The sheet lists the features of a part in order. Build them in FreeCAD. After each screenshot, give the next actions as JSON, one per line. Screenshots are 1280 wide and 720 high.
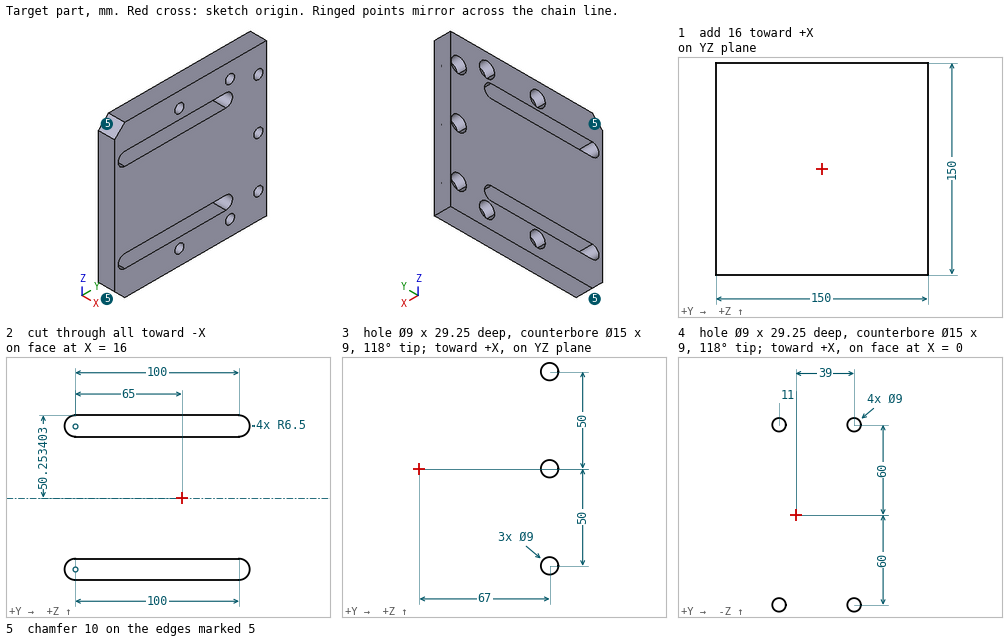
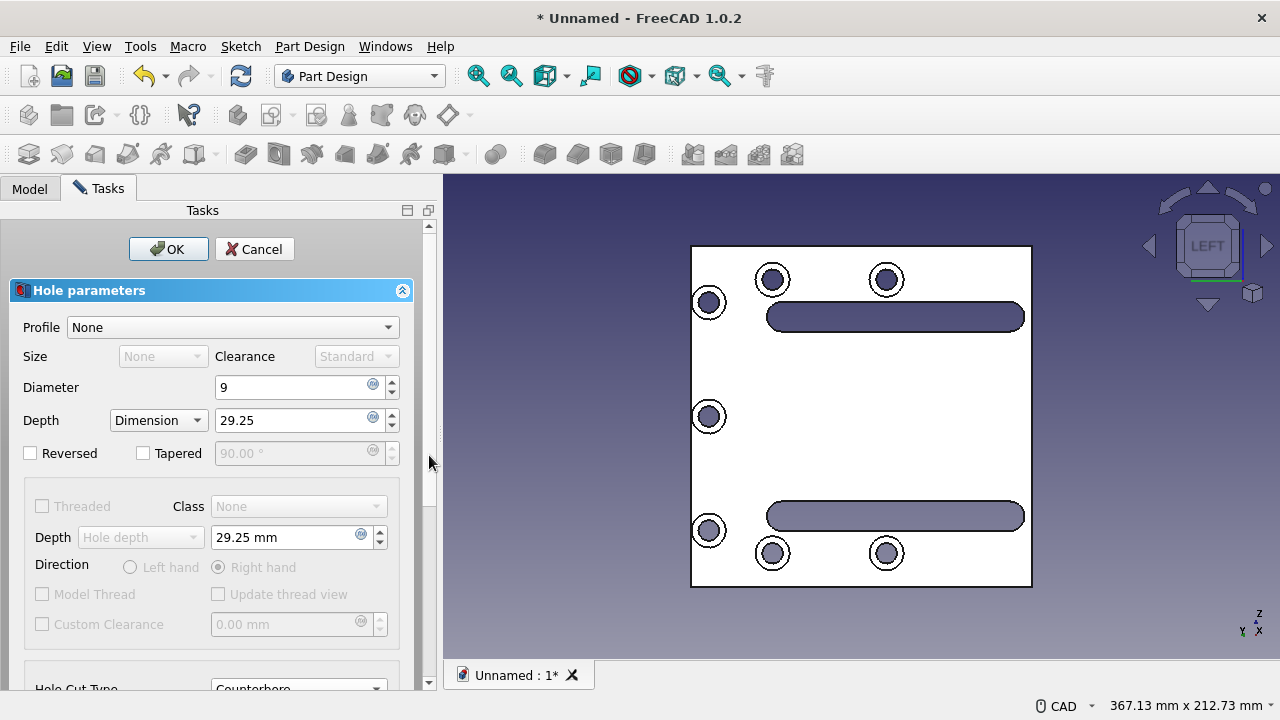
{"action": "left_click", "coordinate": [169, 249]}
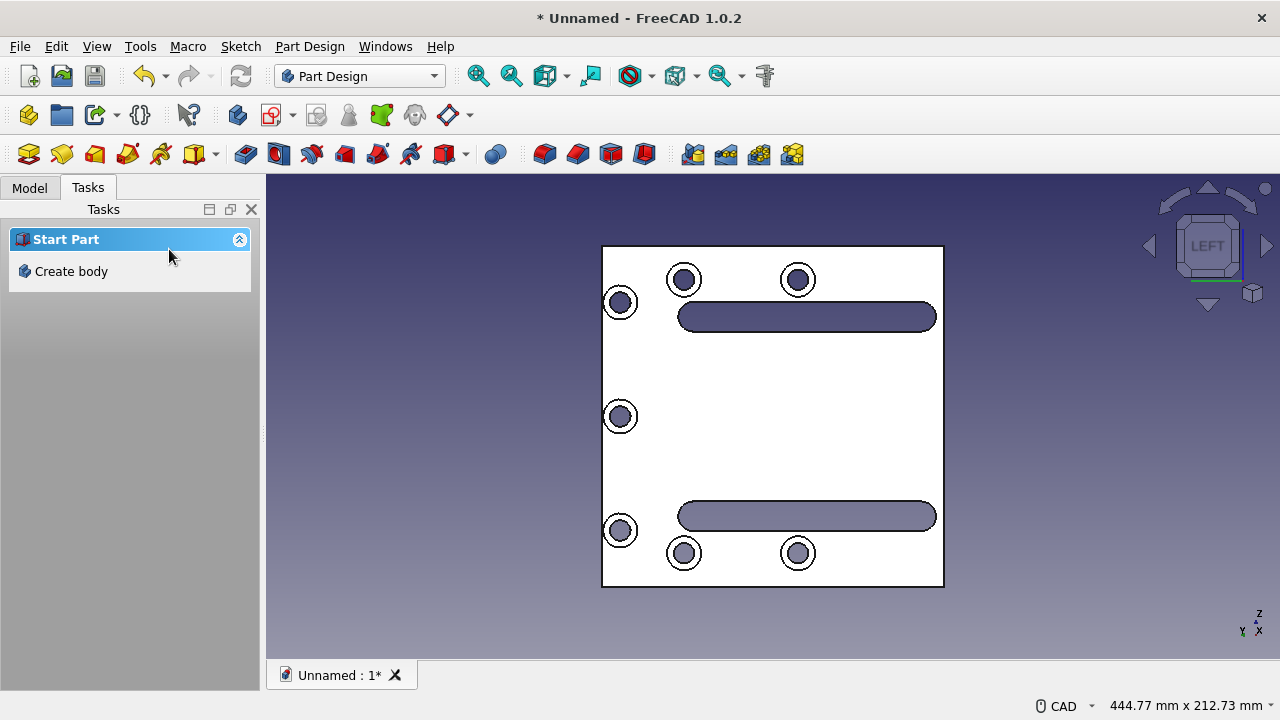
{"action": "key", "text": "0"}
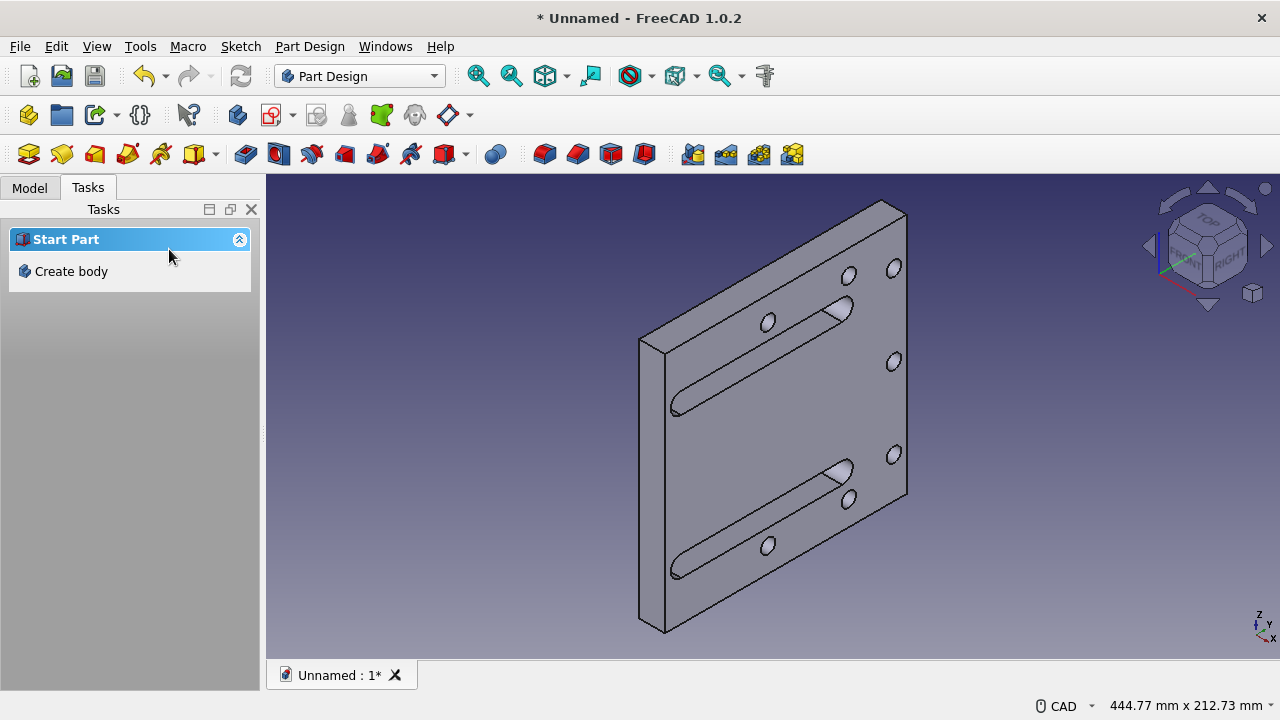
{"action": "left_click", "coordinate": [652, 346]}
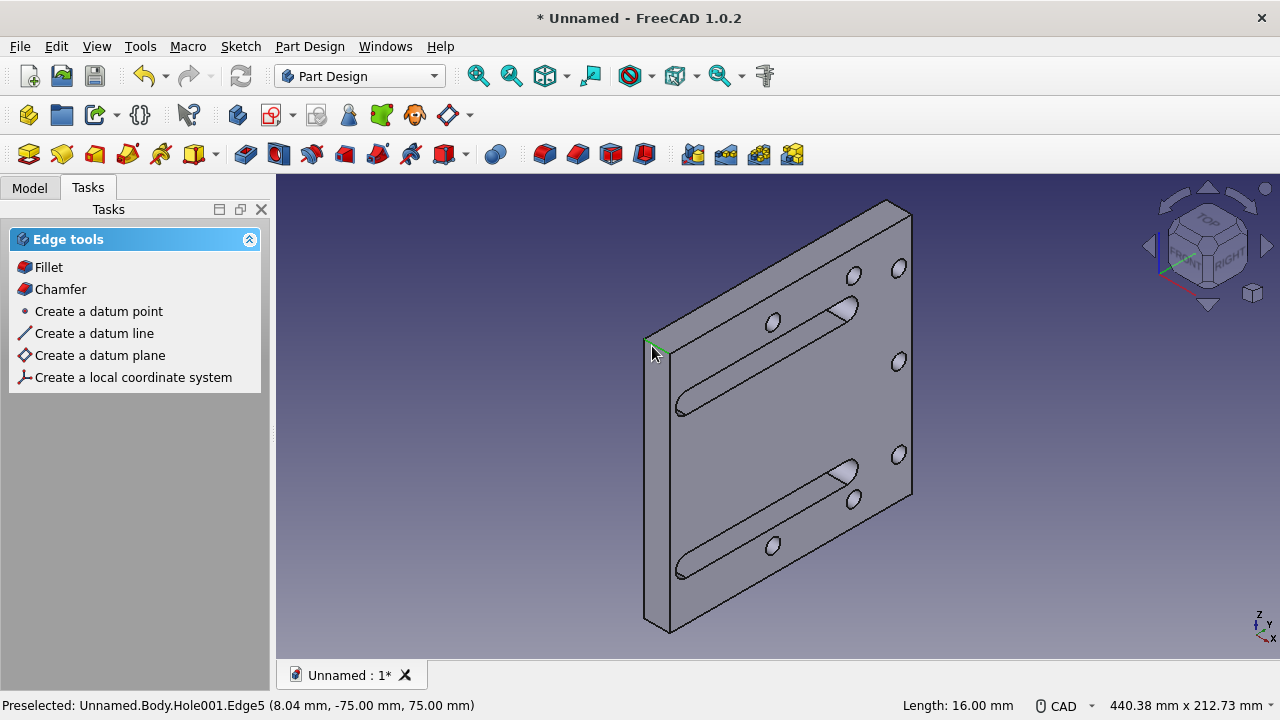
{"action": "key", "text": "2"}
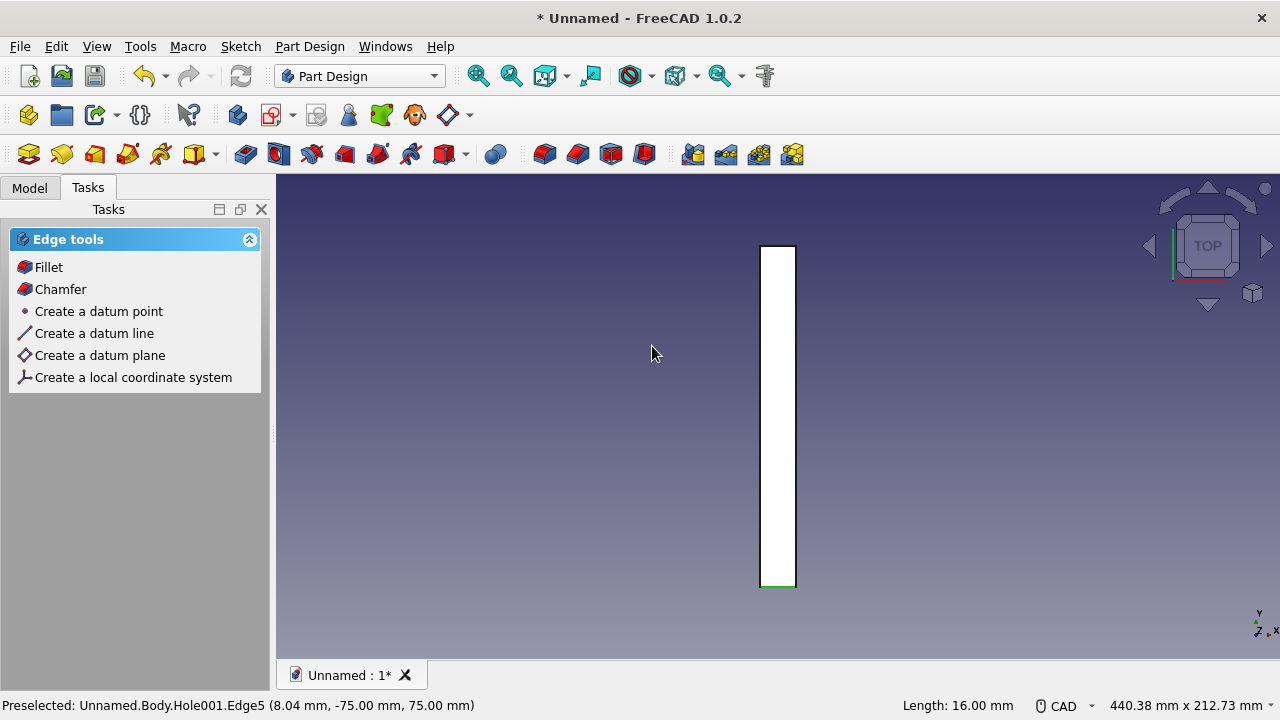
{"action": "key", "text": "1"}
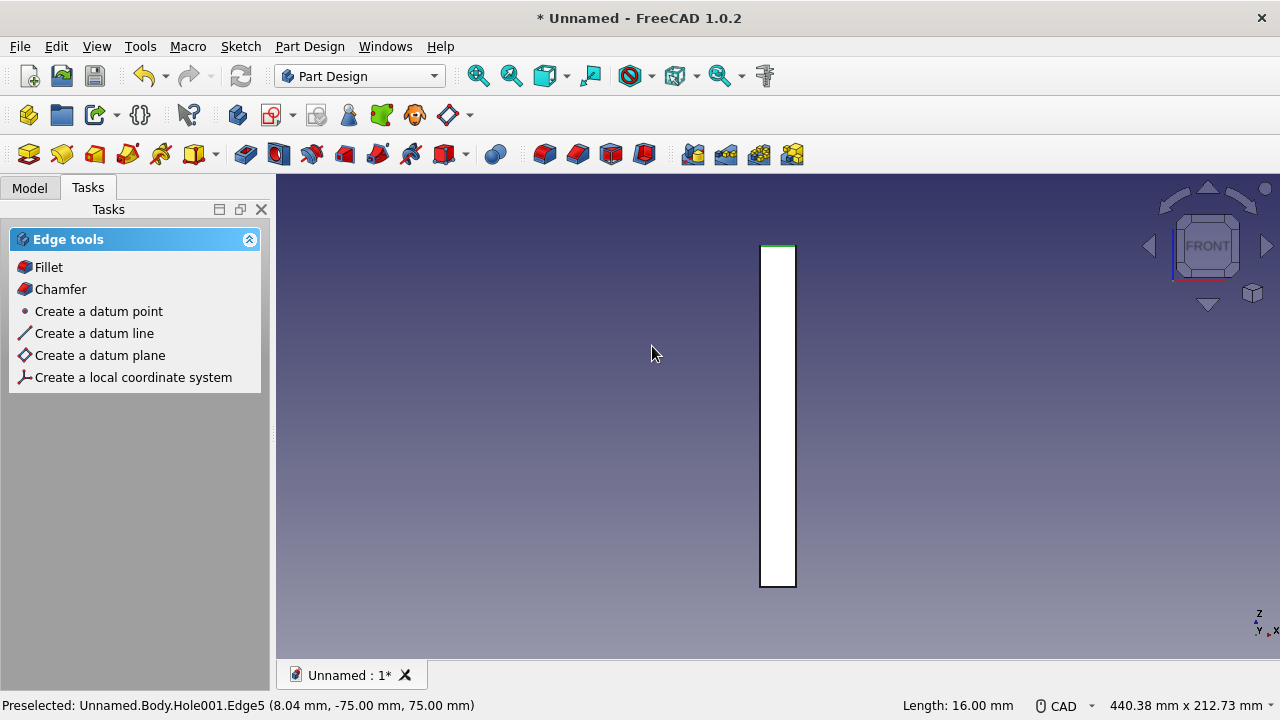
{"action": "left_click", "coordinate": [778, 586], "text": "ctrl"}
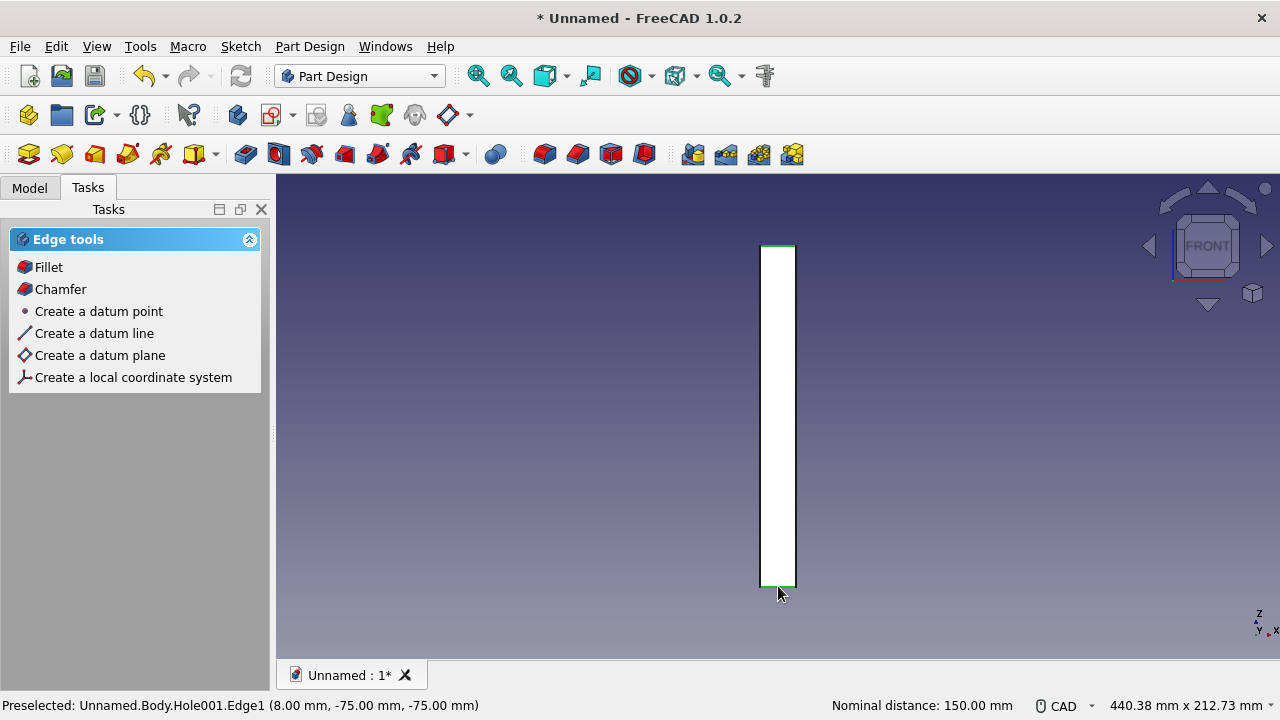
{"action": "left_click", "coordinate": [578, 154]}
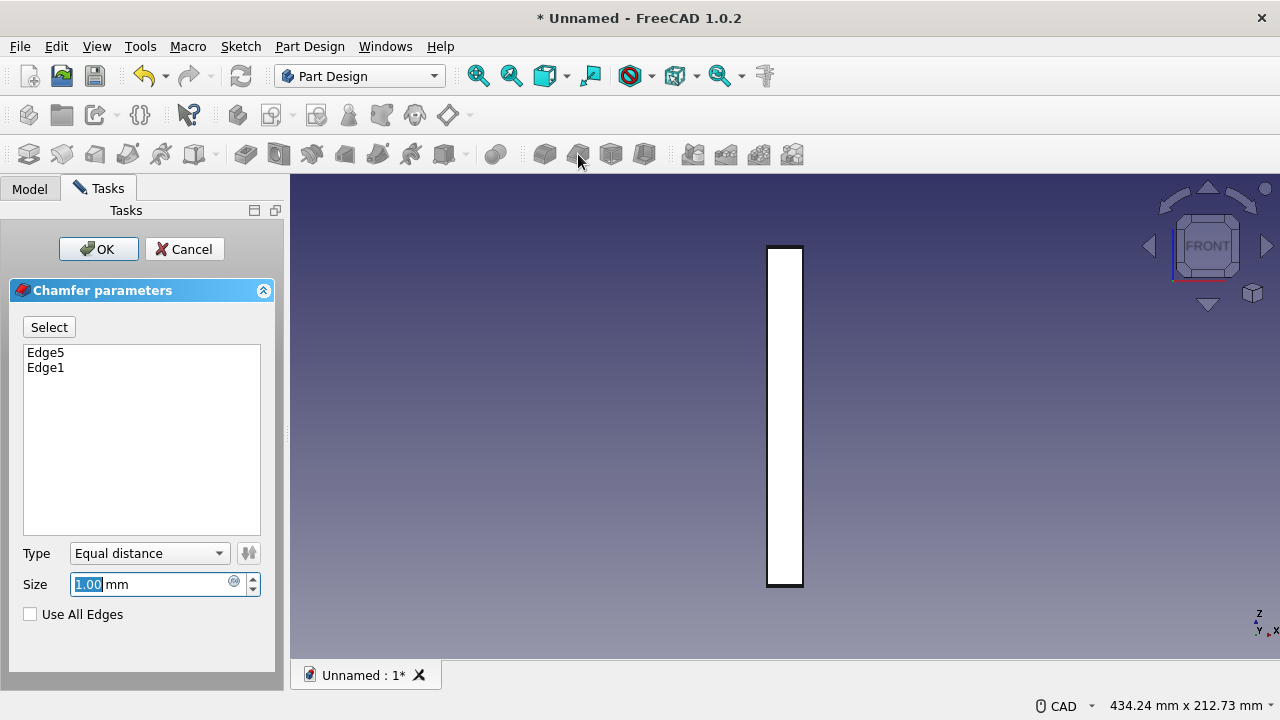
{"action": "type", "text": "10"}
{"action": "key", "text": "Tab"}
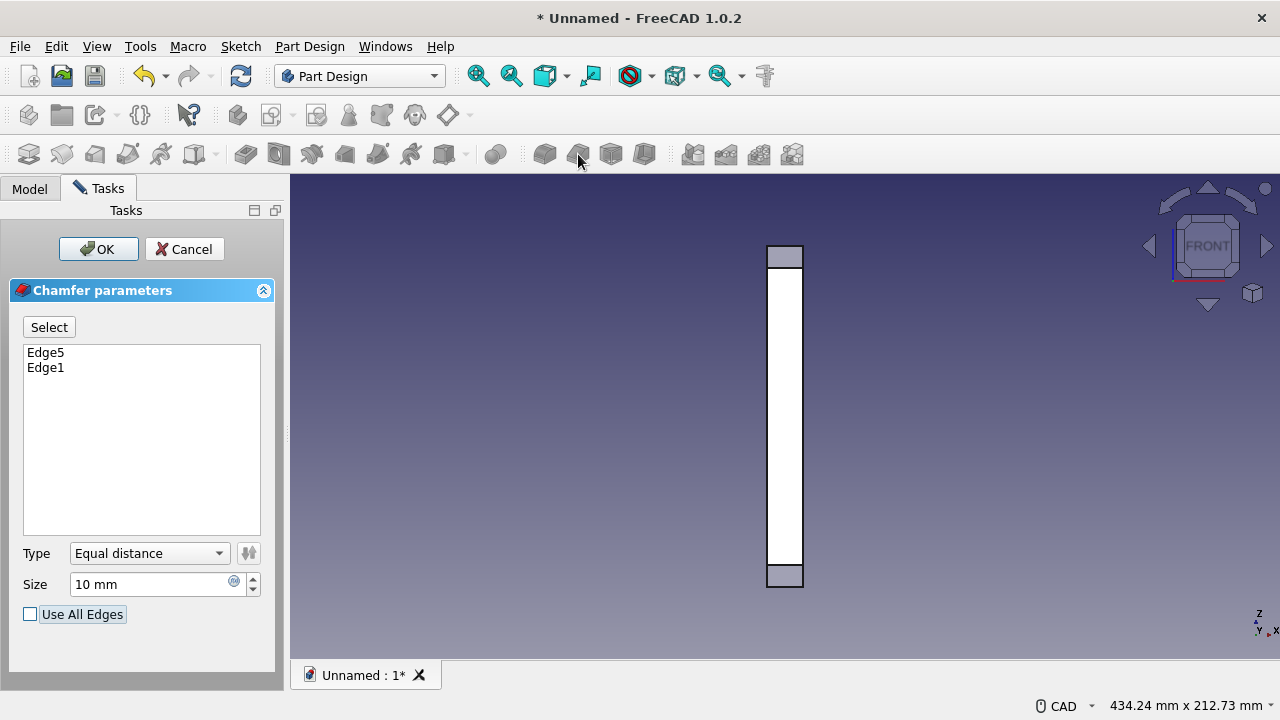
{"action": "left_click", "coordinate": [99, 249]}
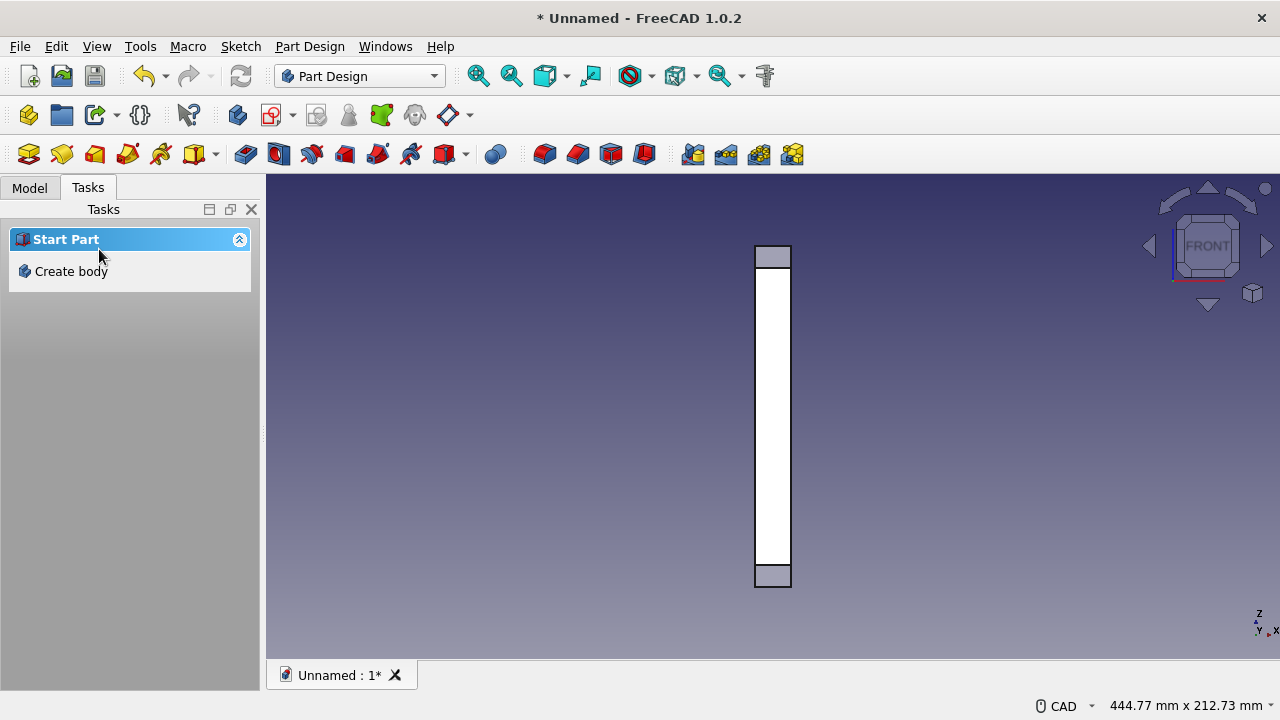
{"action": "key", "text": "0"}